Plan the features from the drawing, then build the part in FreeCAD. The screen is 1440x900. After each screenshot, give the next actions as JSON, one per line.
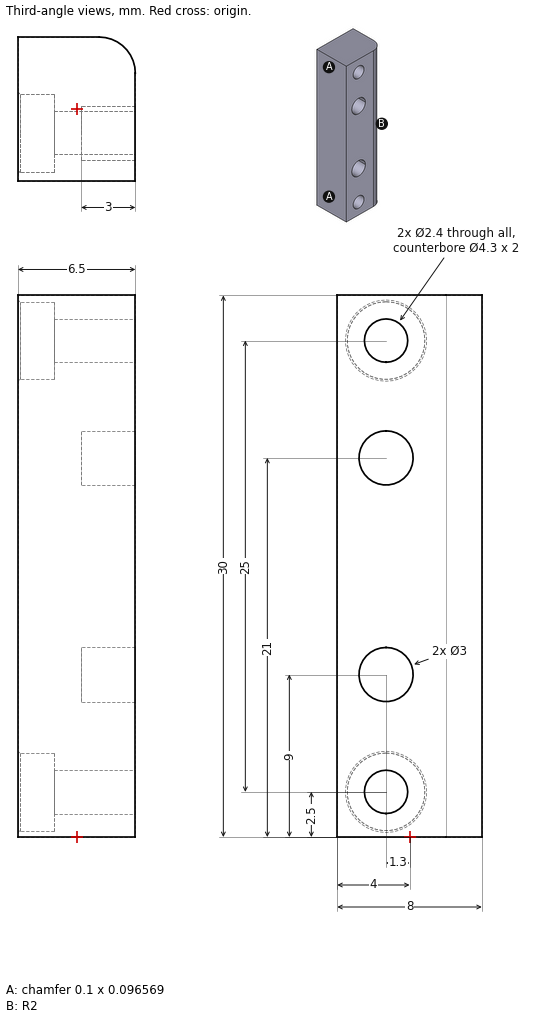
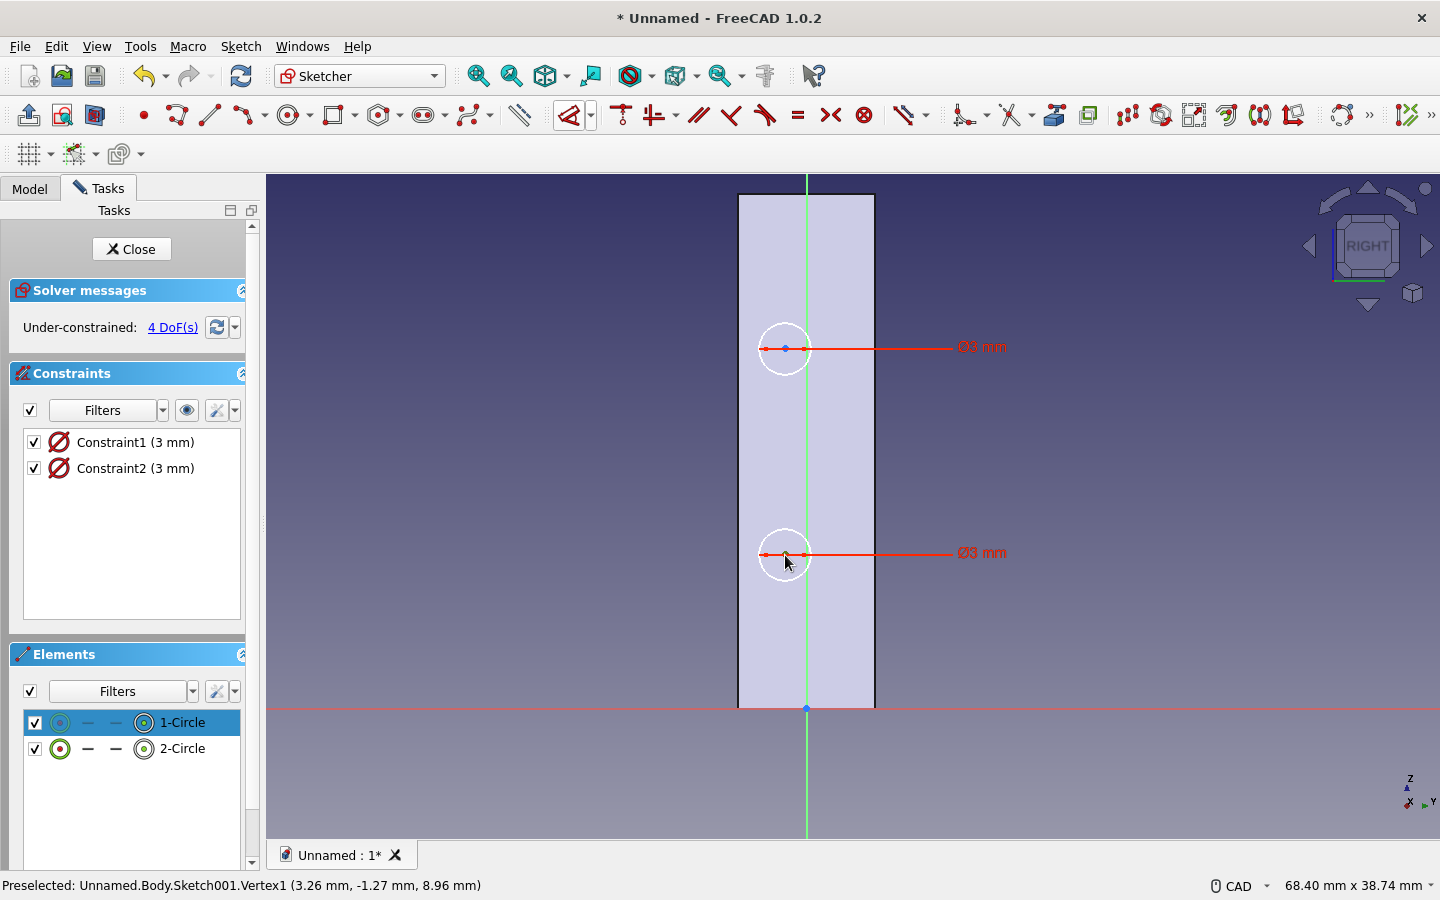
{"action": "left_click", "coordinate": [785, 349]}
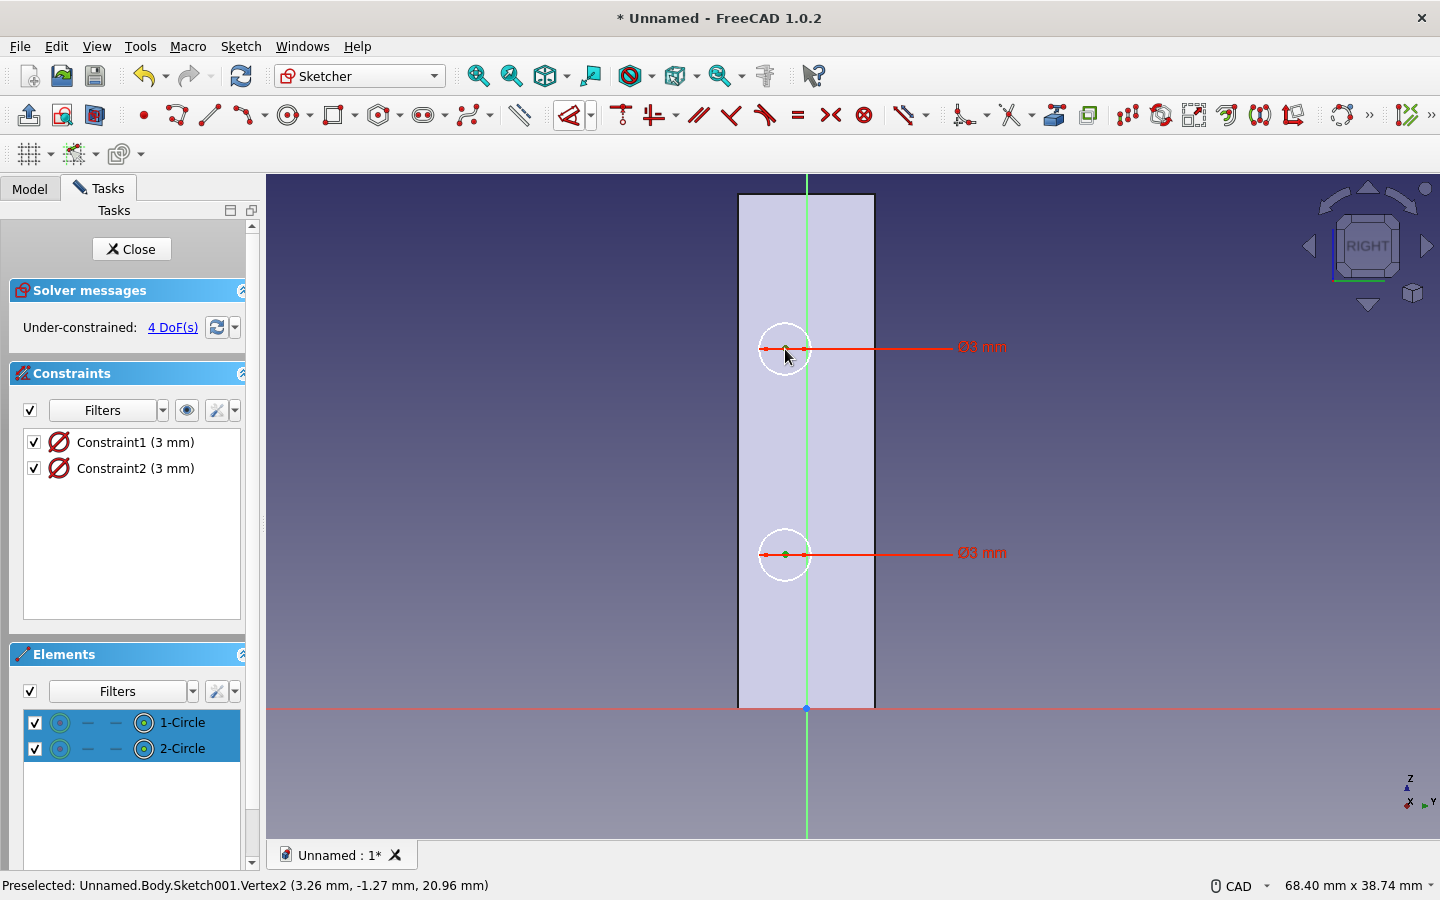
{"action": "left_click", "coordinate": [676, 116]}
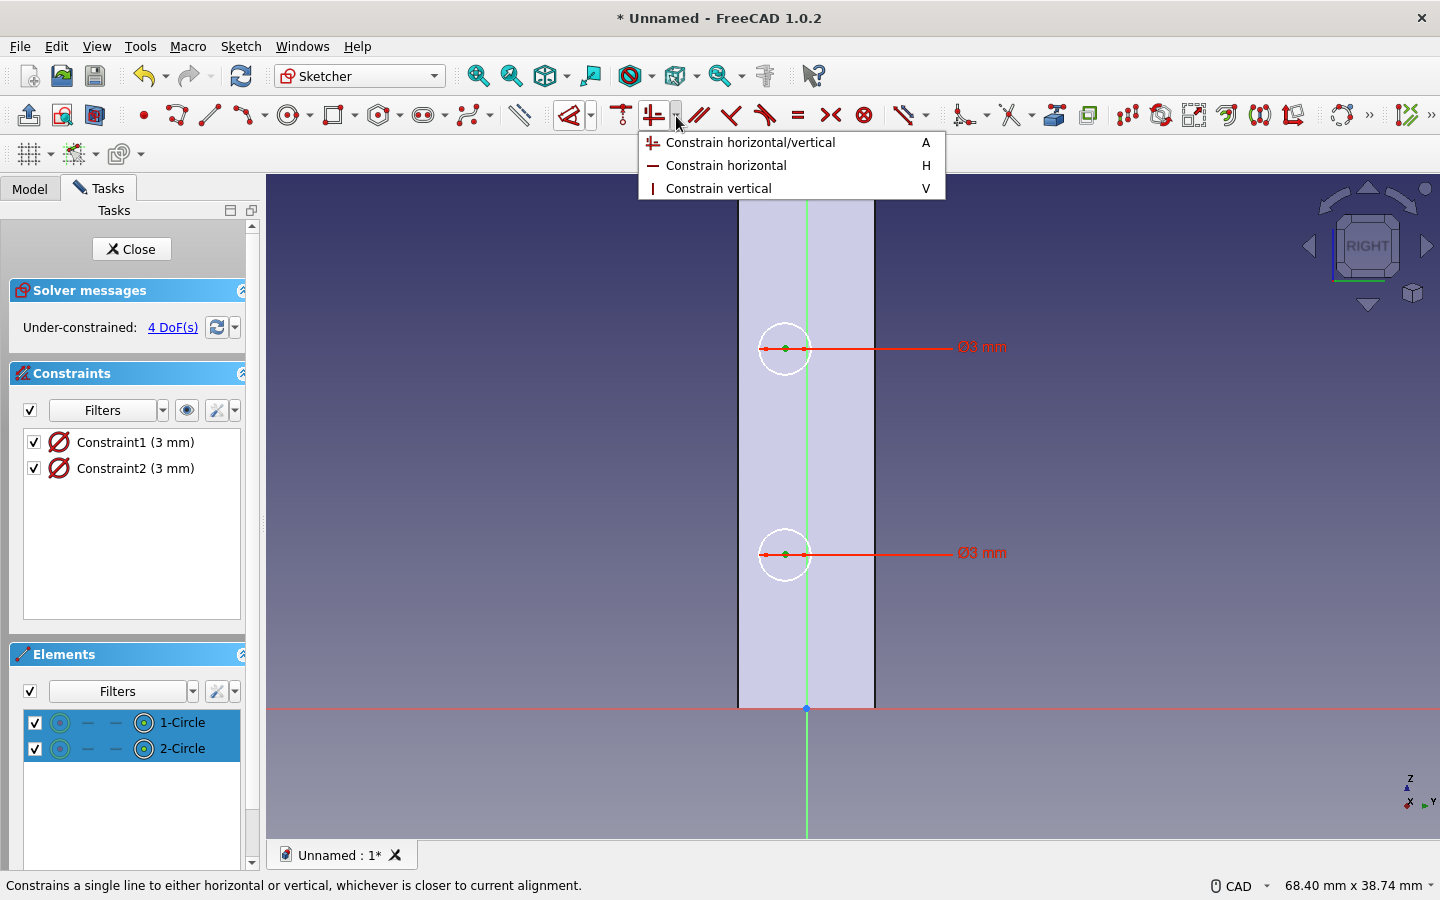
{"action": "left_click", "coordinate": [792, 188]}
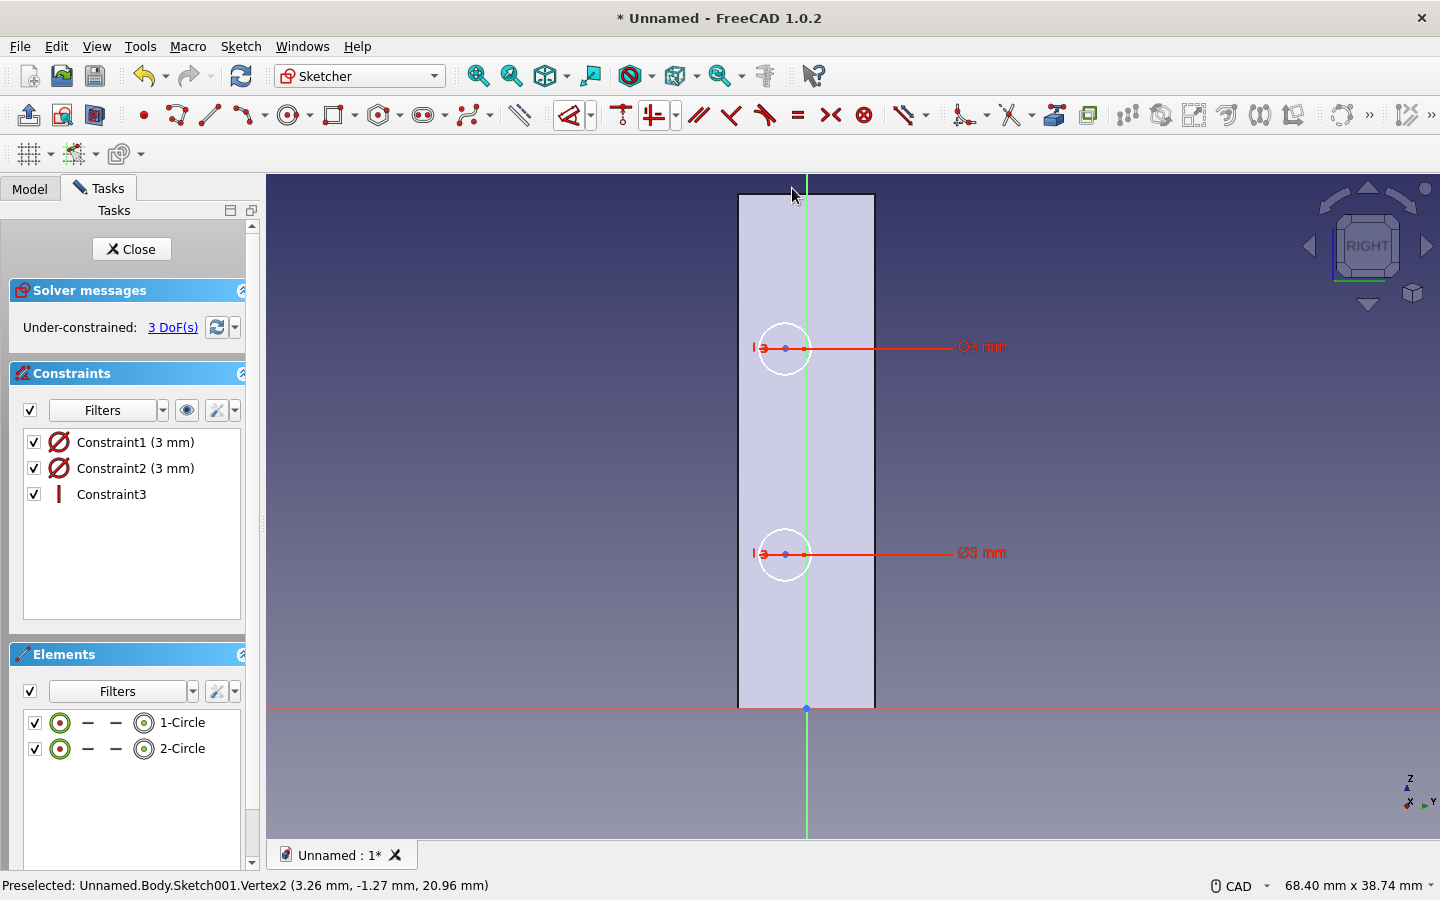
{"action": "left_click", "coordinate": [785, 555]}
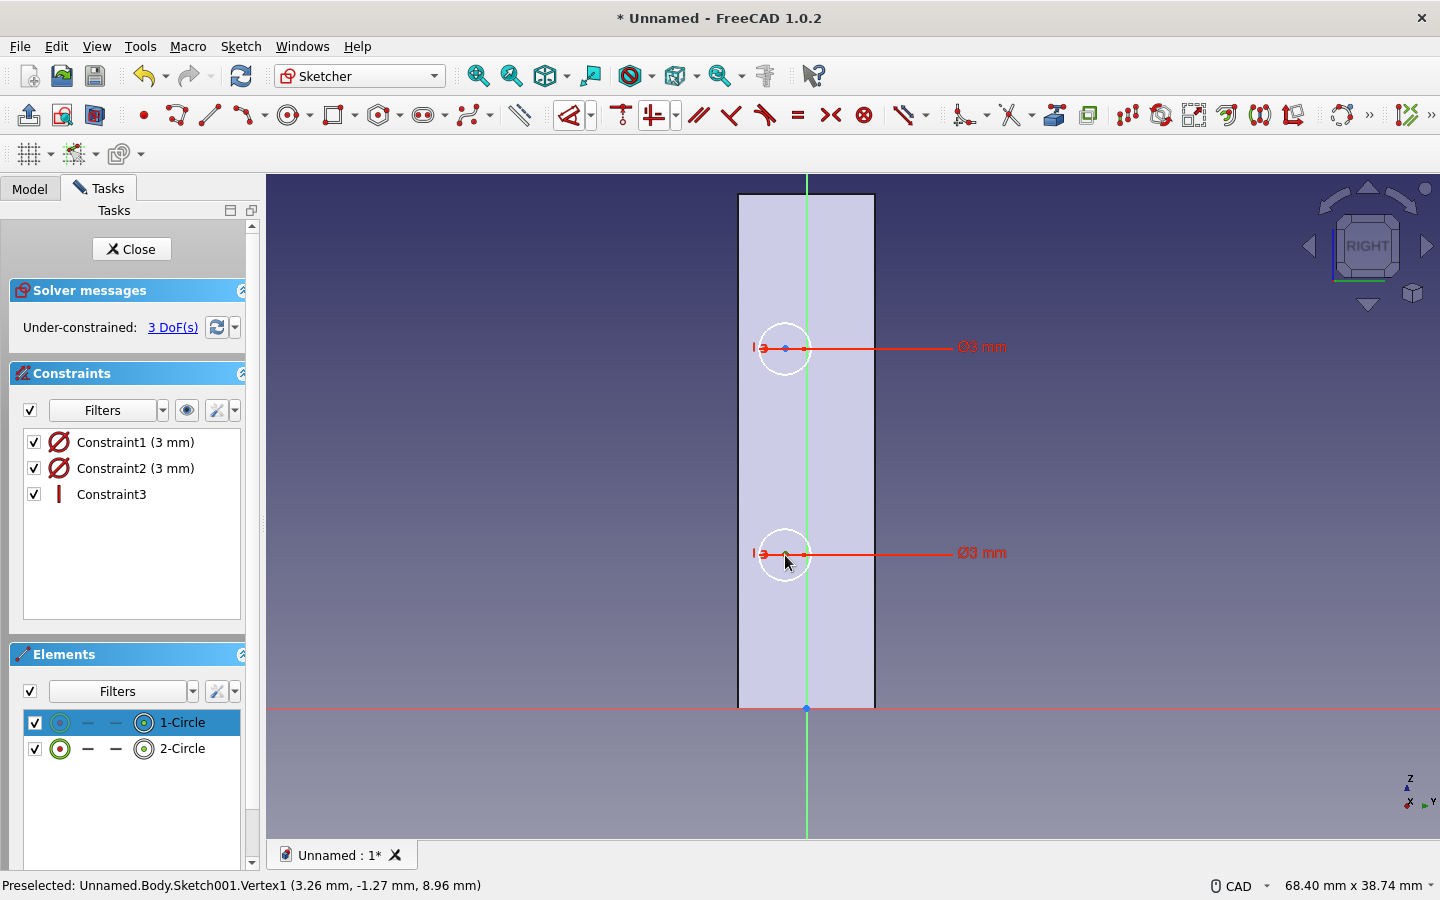
{"action": "left_click", "coordinate": [590, 116]}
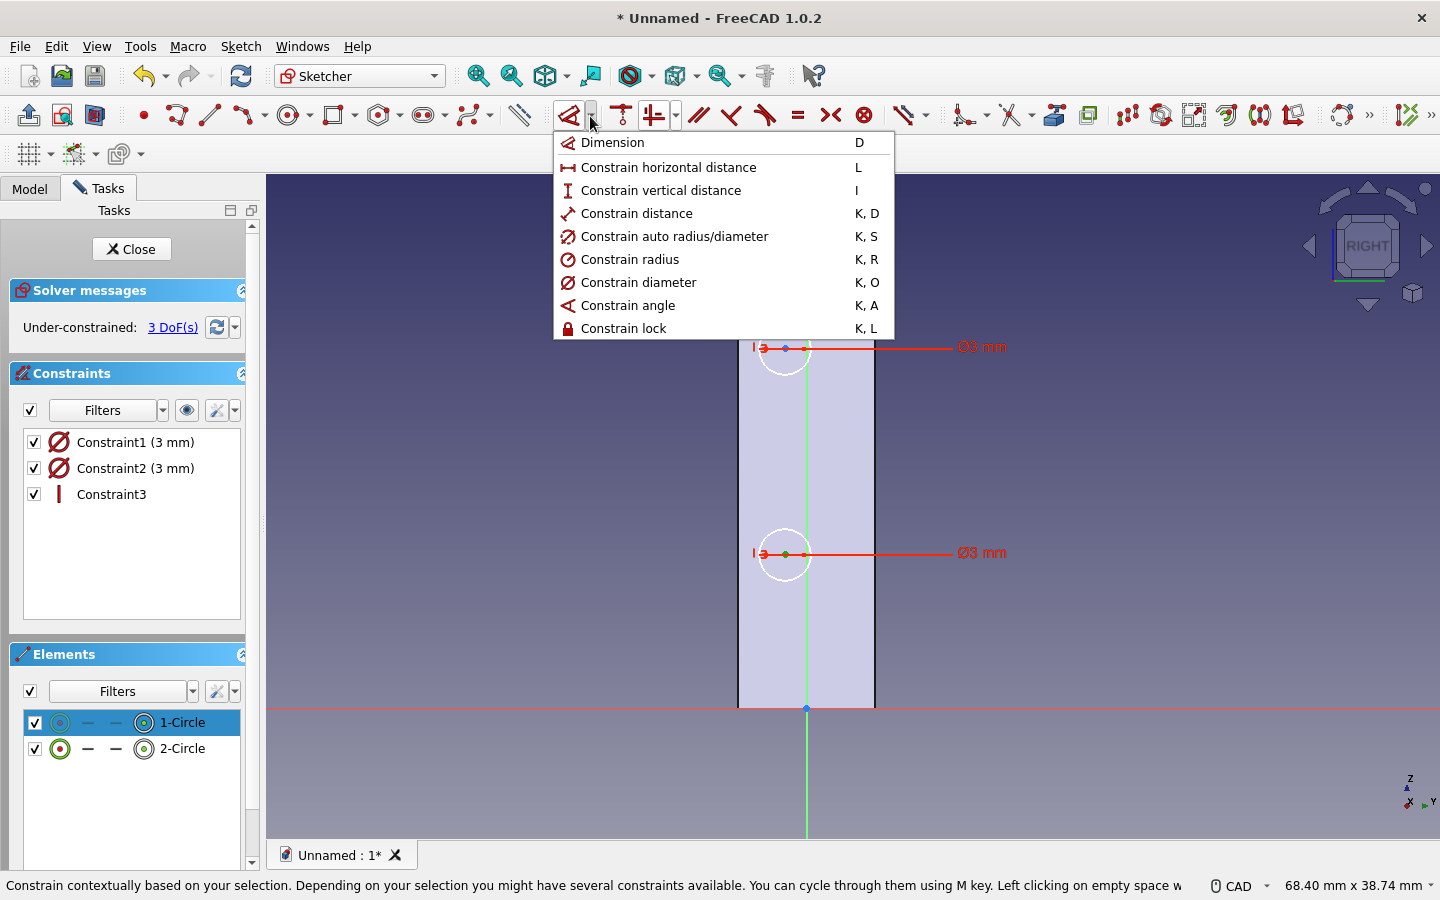
{"action": "left_click", "coordinate": [724, 190]}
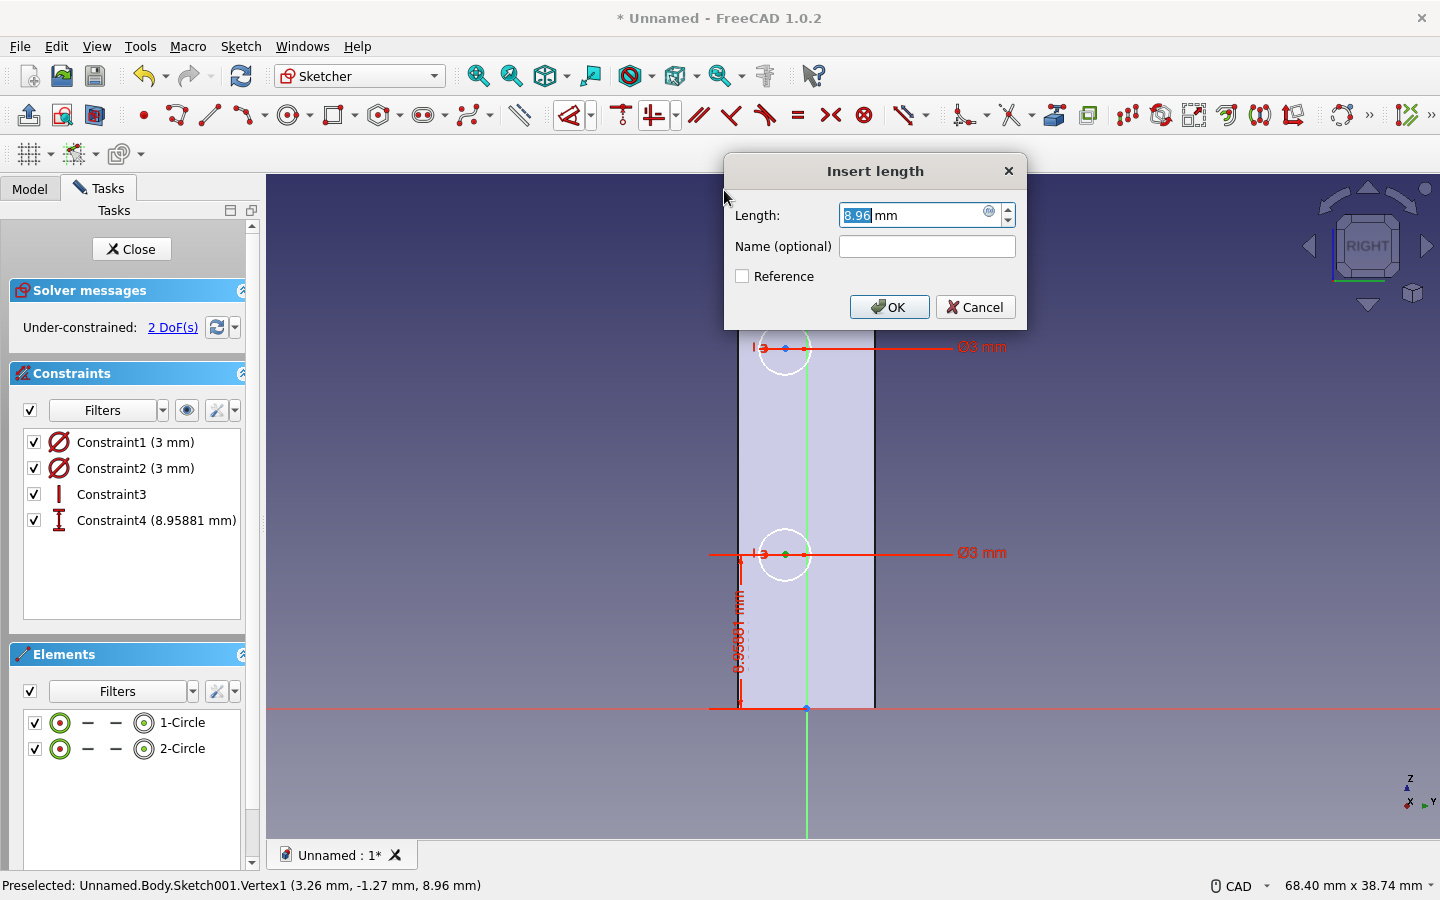
{"action": "type", "text": "9"}
{"action": "key", "text": "Return"}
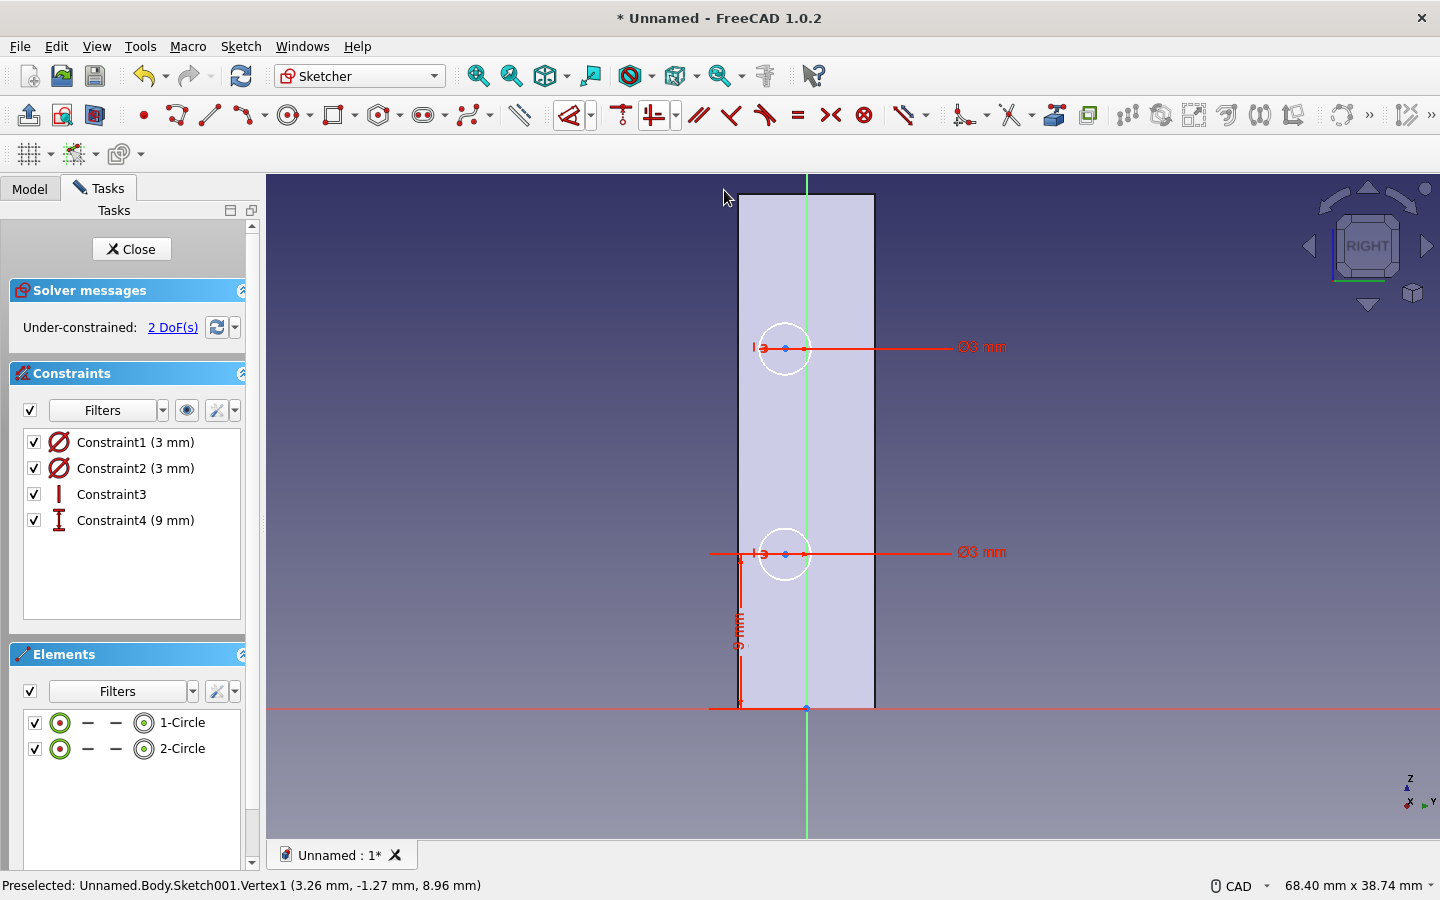
{"action": "left_click", "coordinate": [785, 349]}